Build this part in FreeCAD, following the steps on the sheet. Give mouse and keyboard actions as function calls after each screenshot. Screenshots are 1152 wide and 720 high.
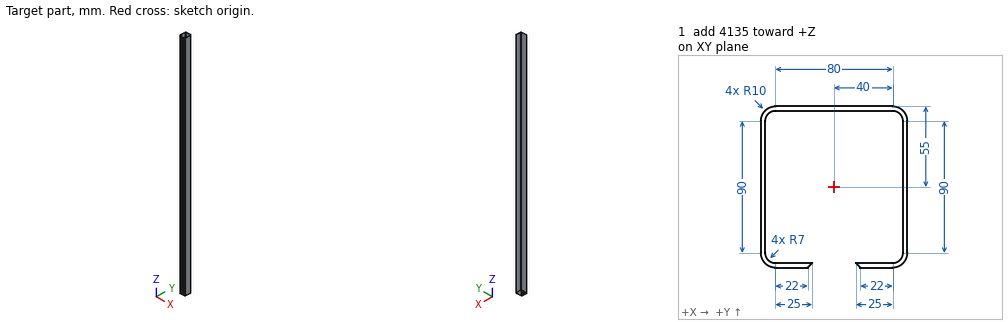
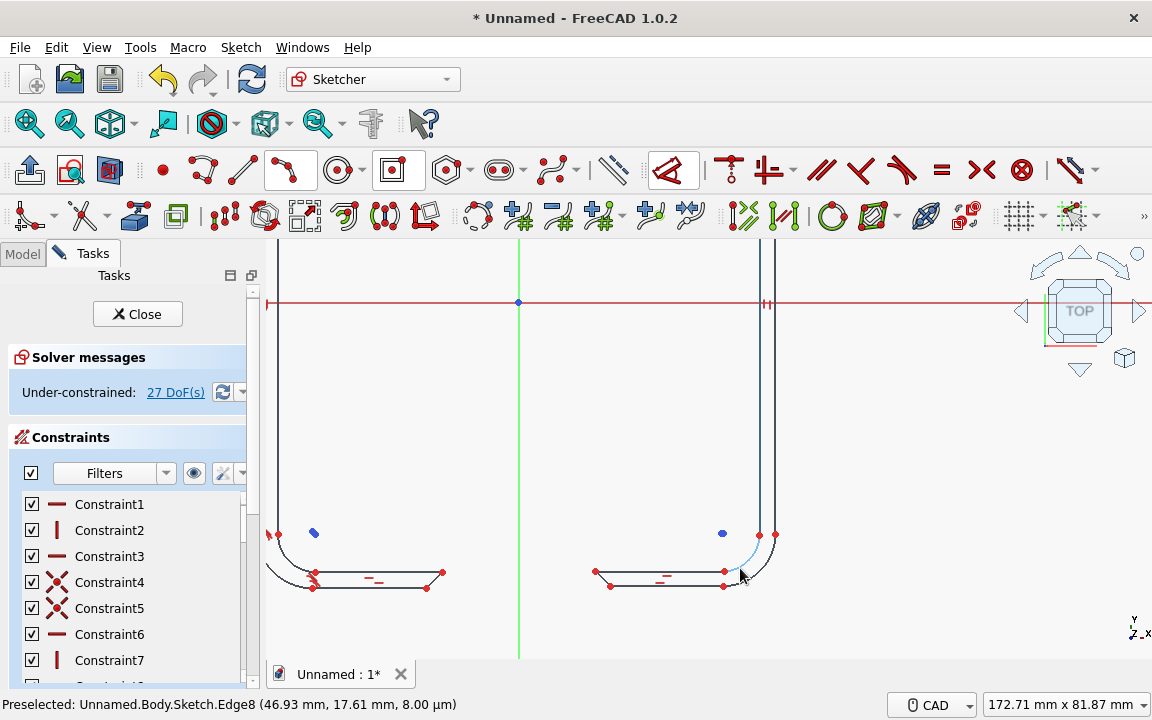
click(740, 567)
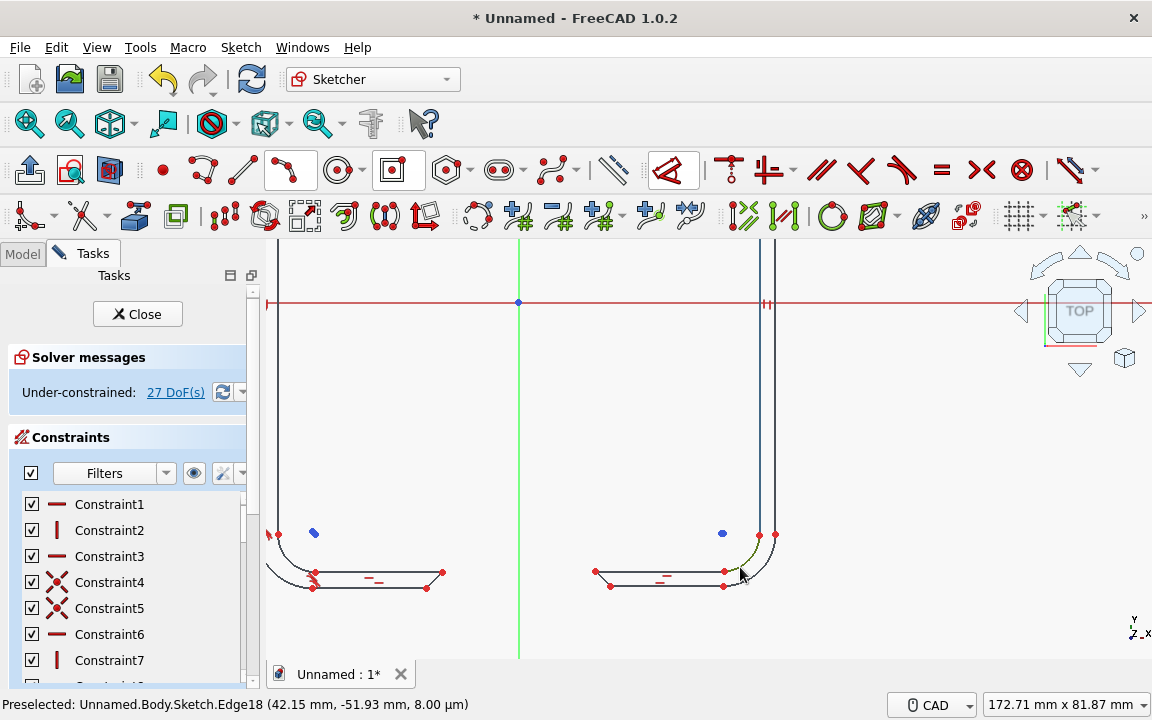
click(902, 170)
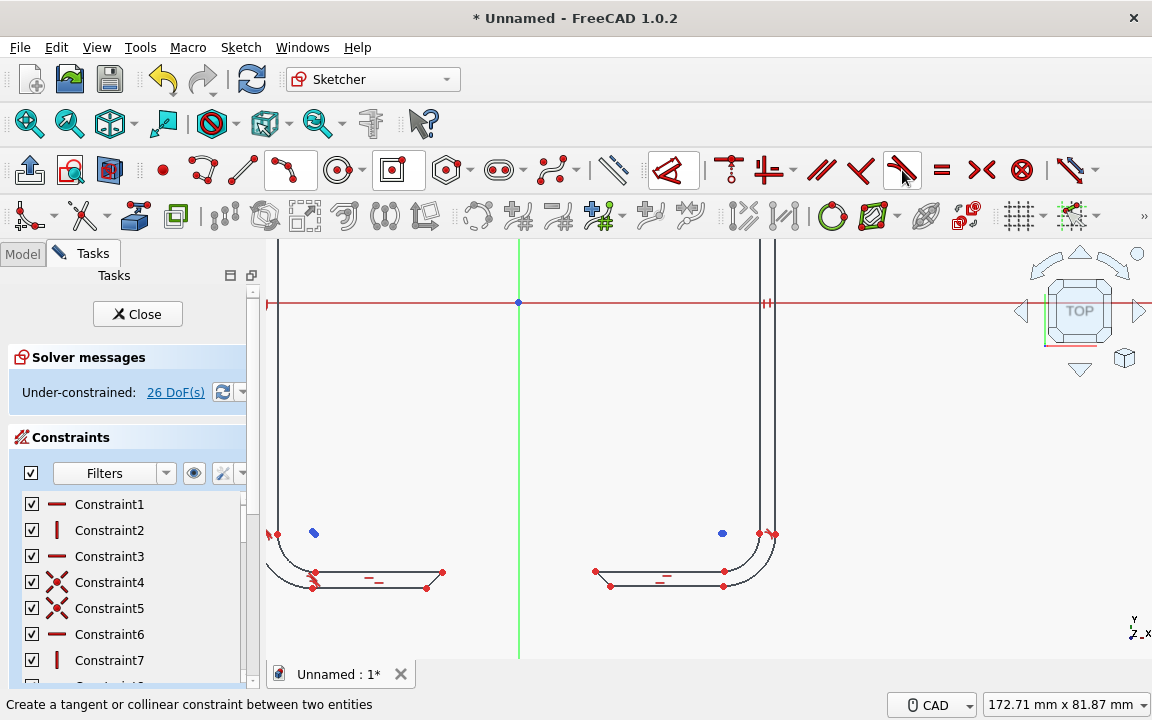
click(686, 572)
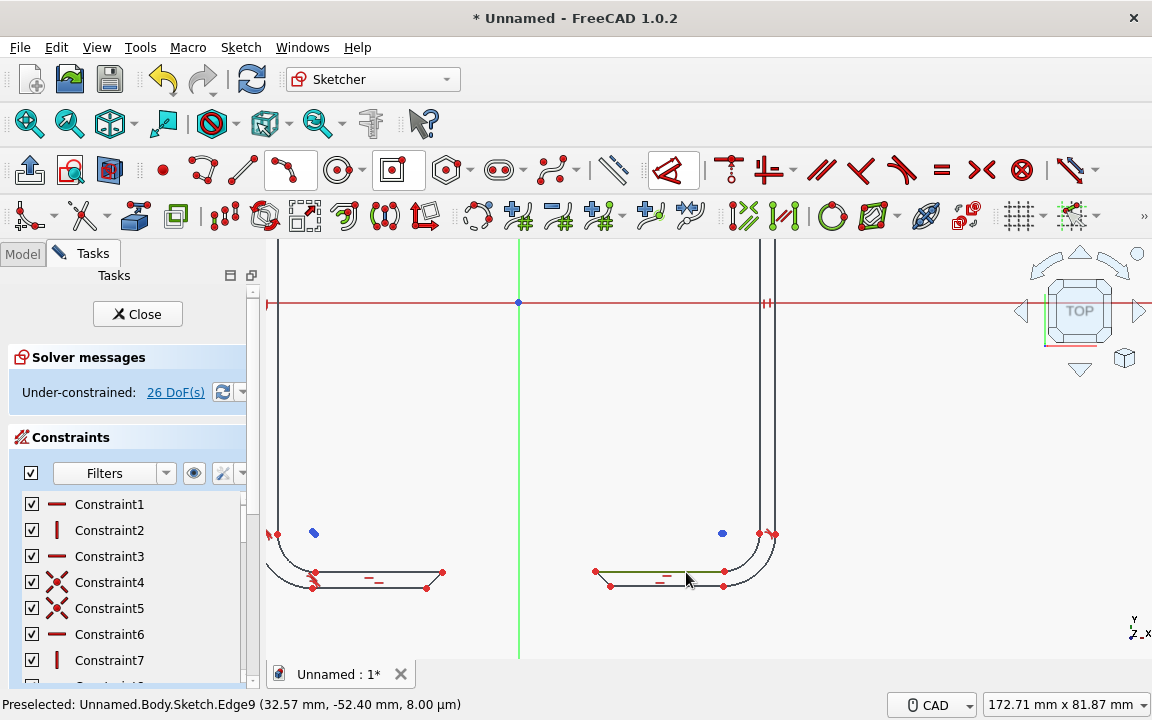
click(741, 566)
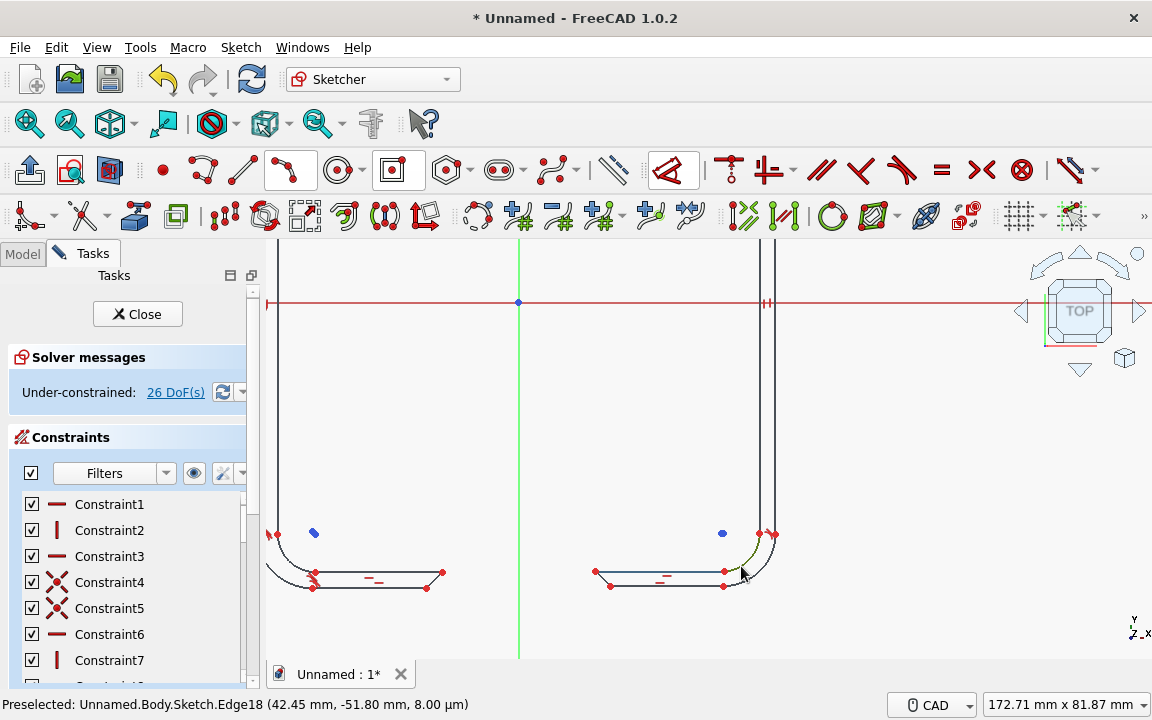
click(902, 170)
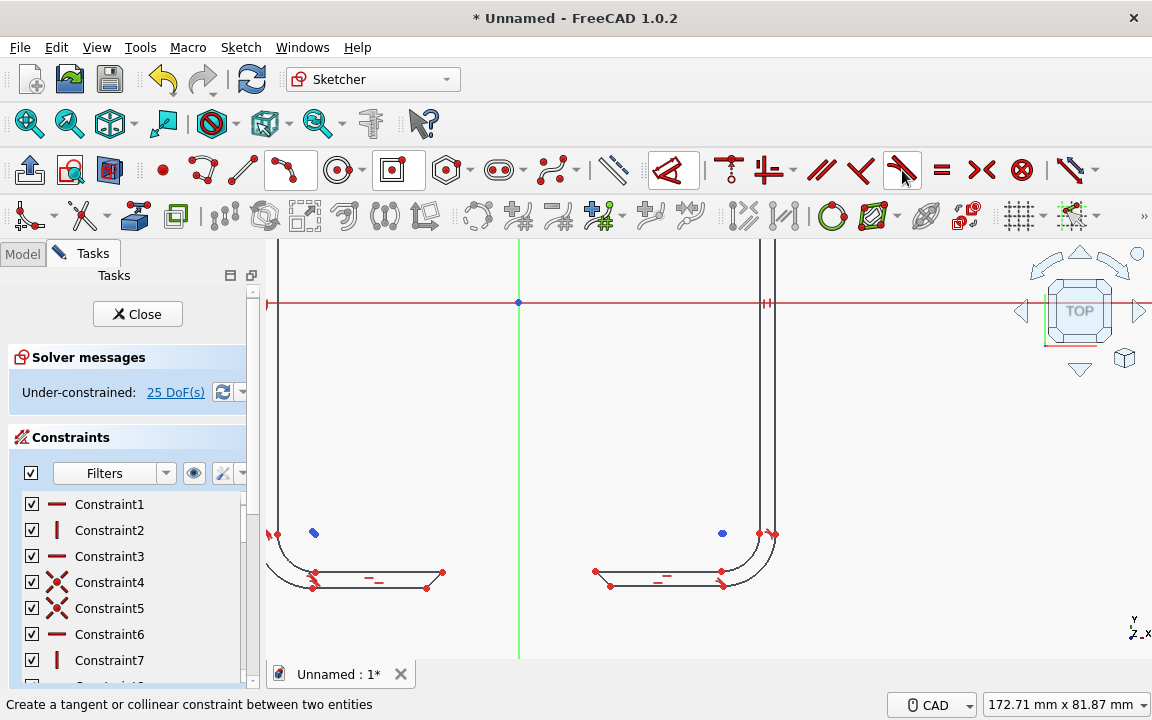
click(645, 586)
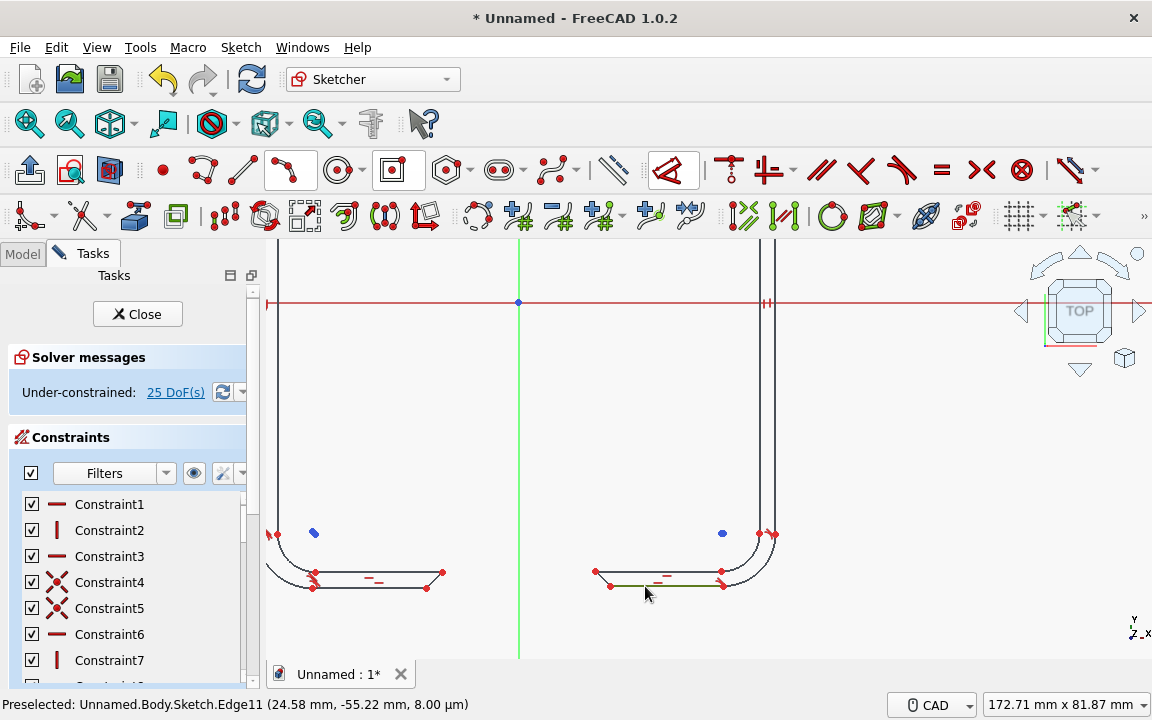
click(747, 580)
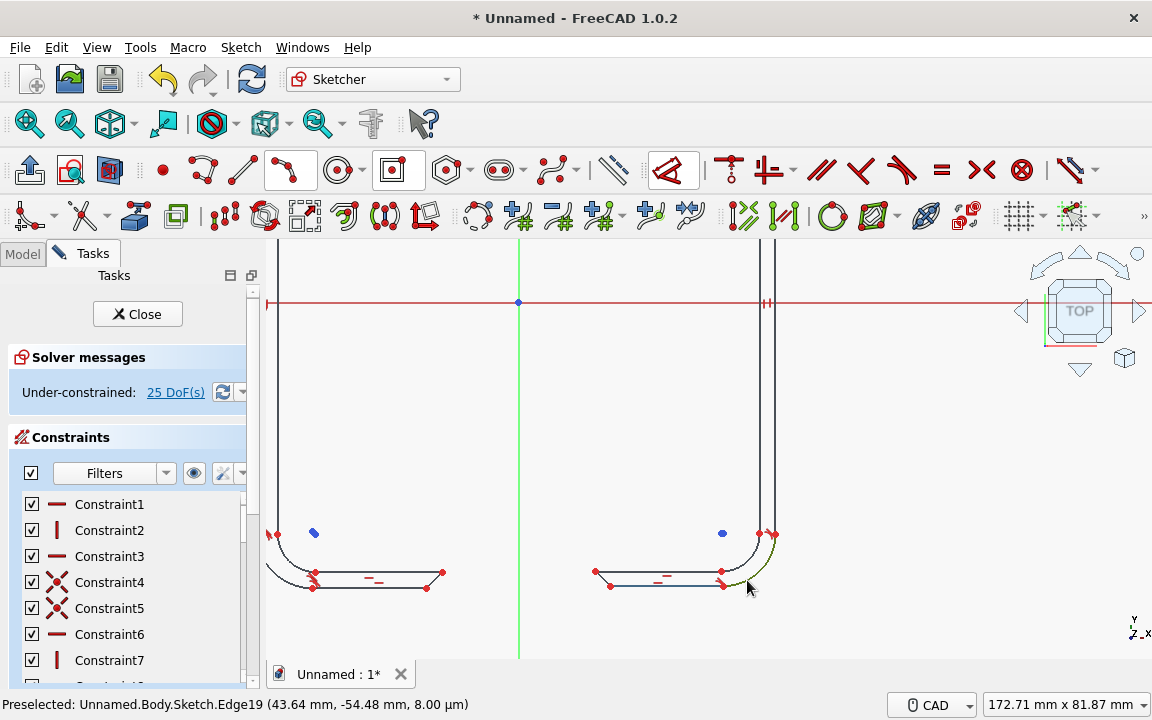
click(902, 170)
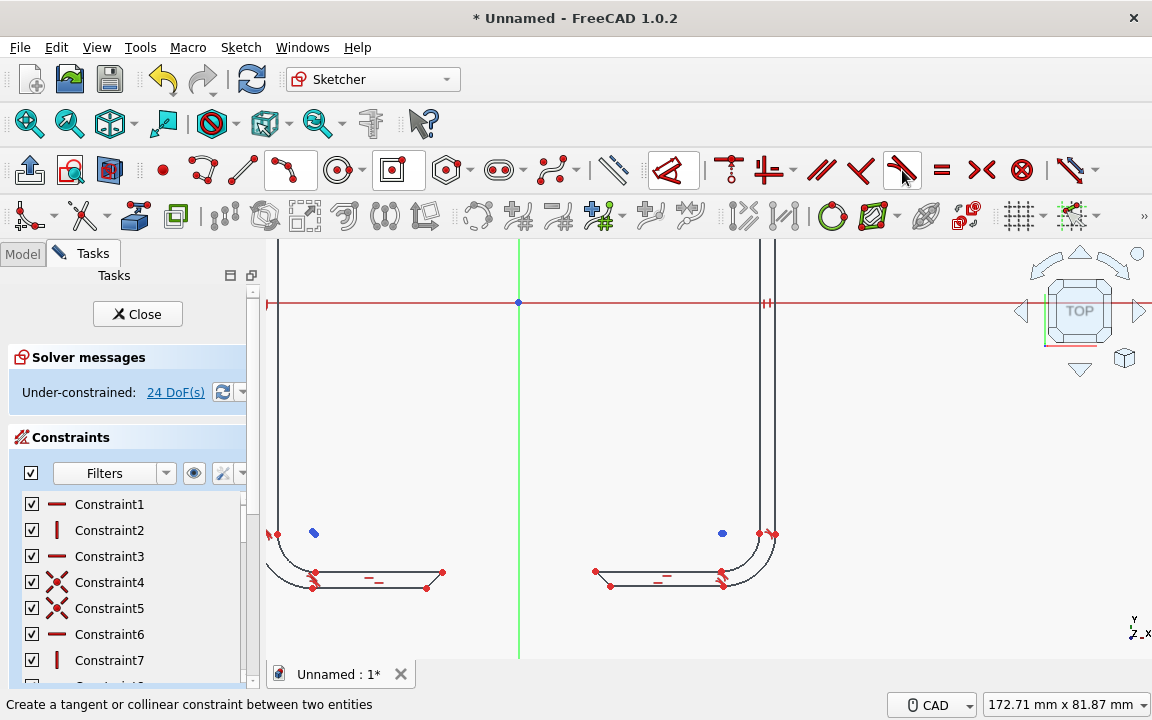
click(775, 396)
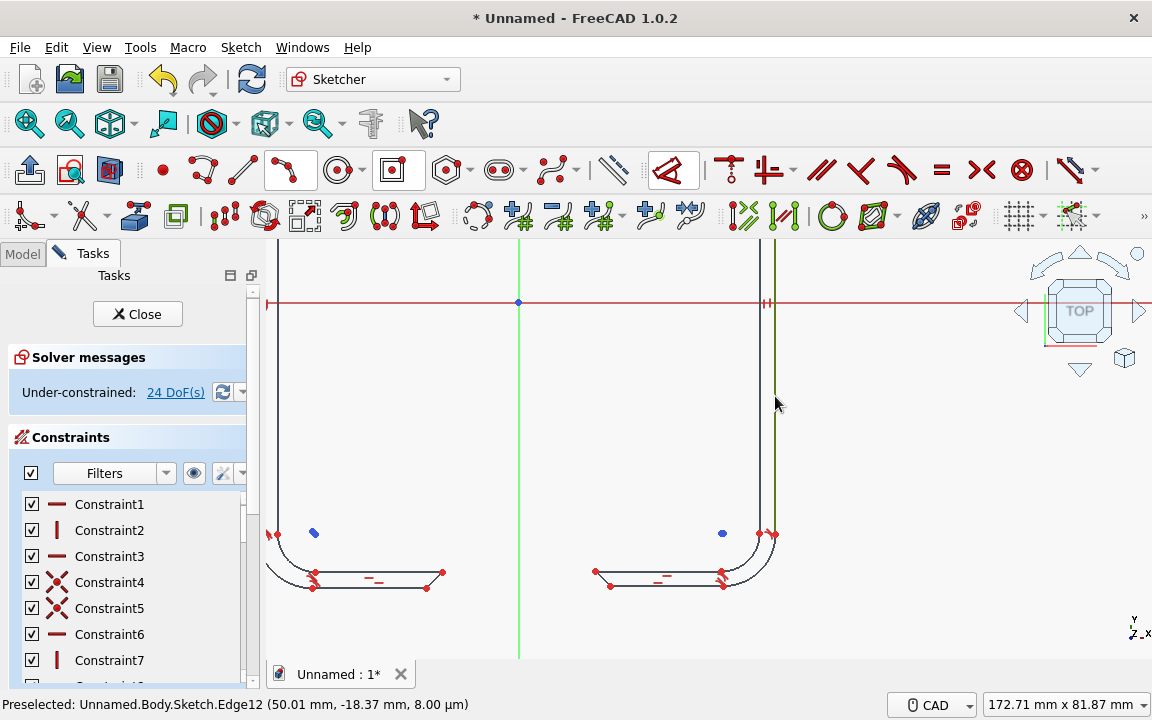
click(747, 580)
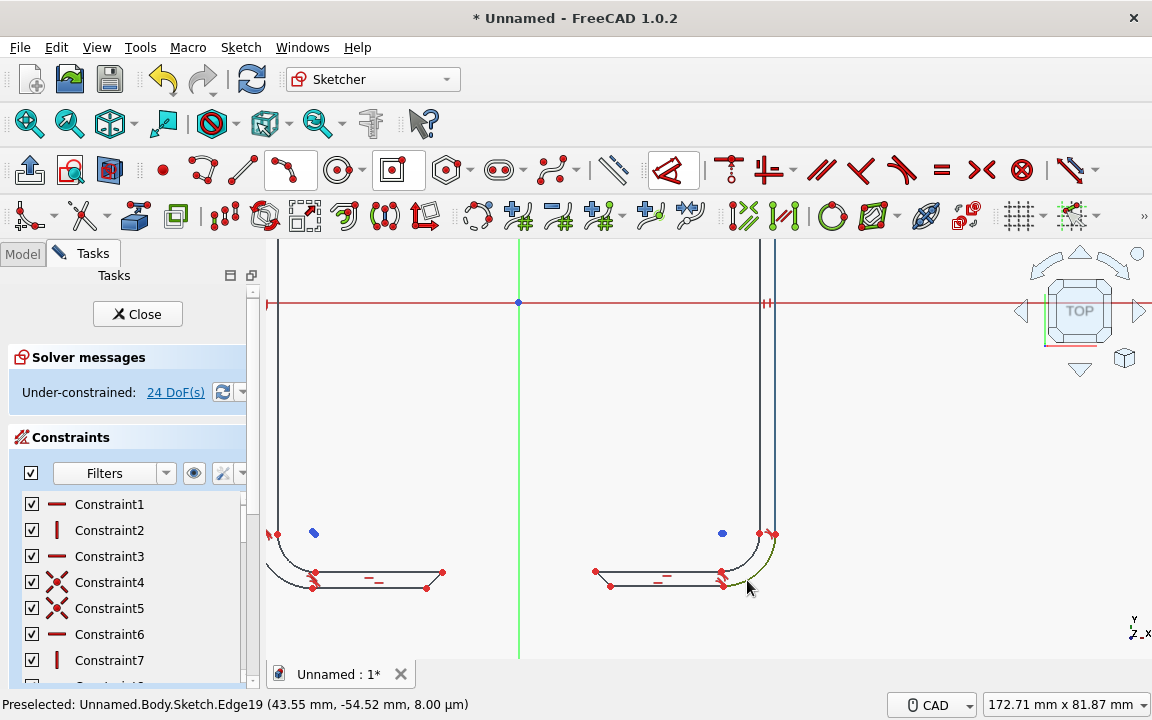
click(902, 170)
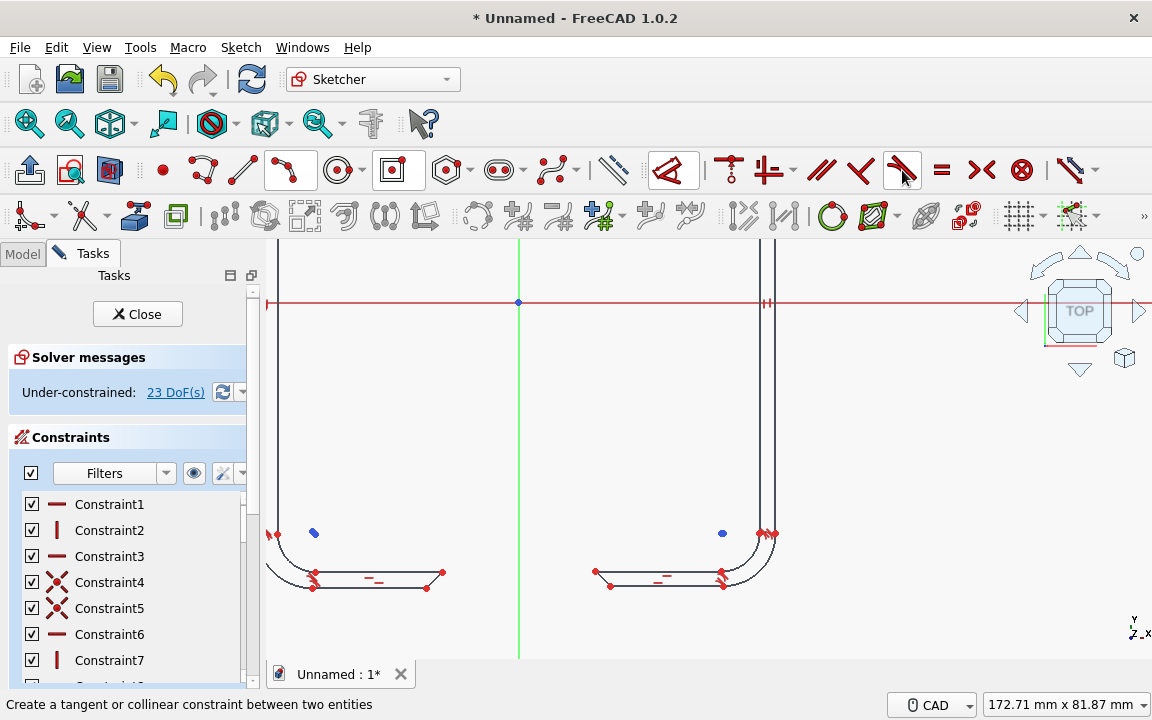
click(775, 395)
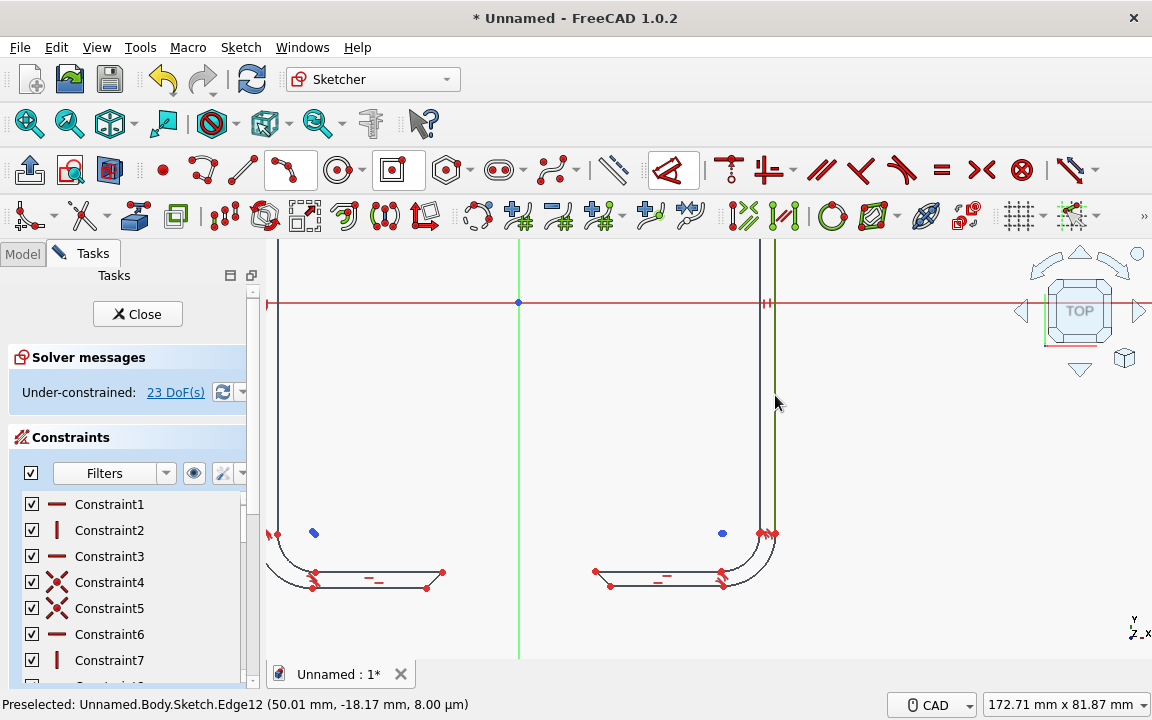
scroll(740, 568, down, 4)